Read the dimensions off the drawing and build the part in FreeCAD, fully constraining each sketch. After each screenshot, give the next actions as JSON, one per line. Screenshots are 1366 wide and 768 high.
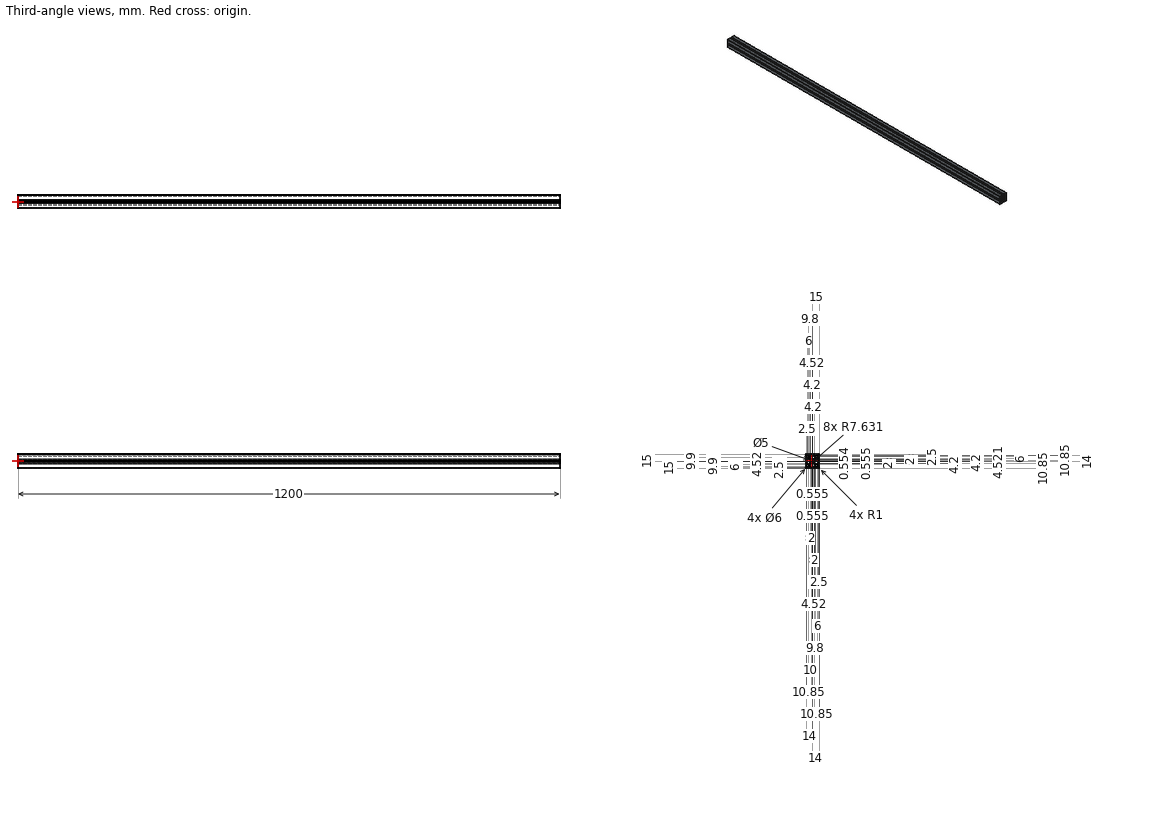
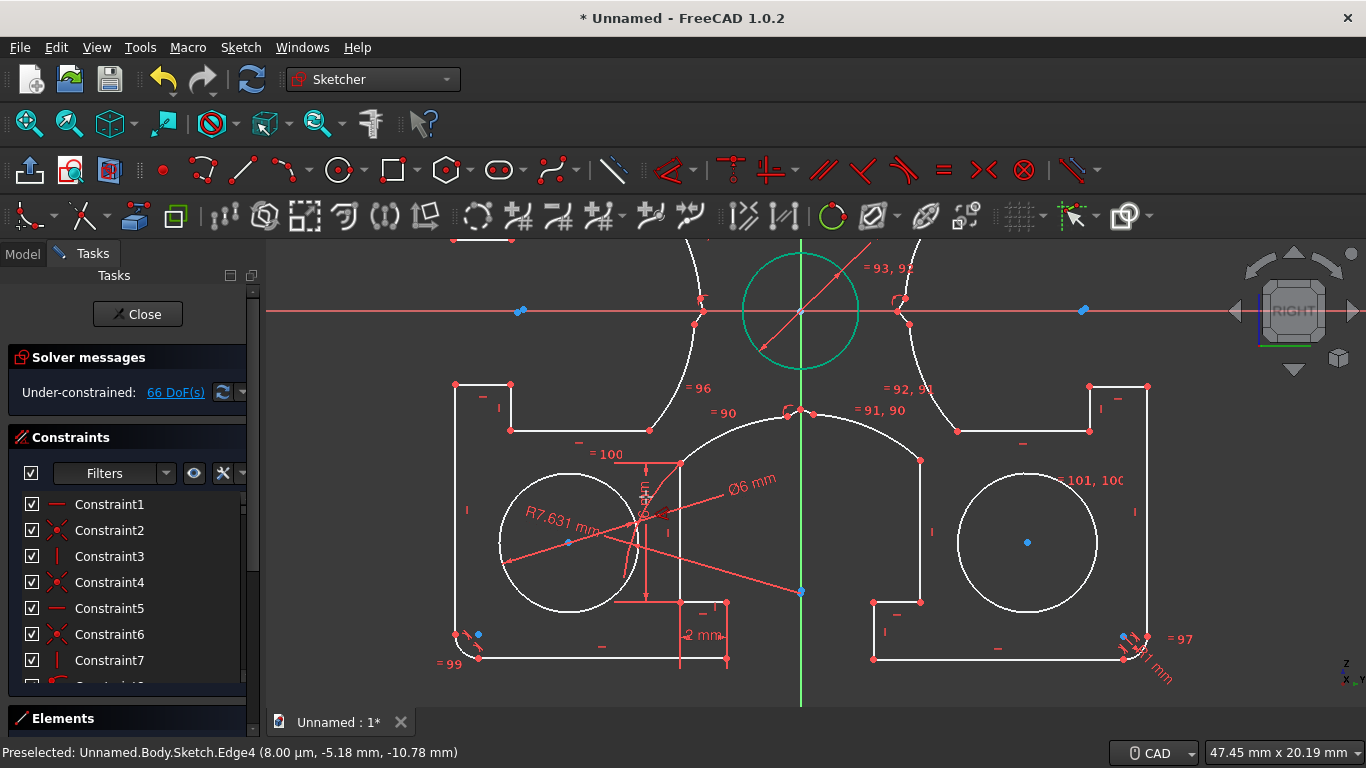
{"action": "left_click", "coordinate": [920, 503]}
{"action": "left_click", "coordinate": [954, 499]}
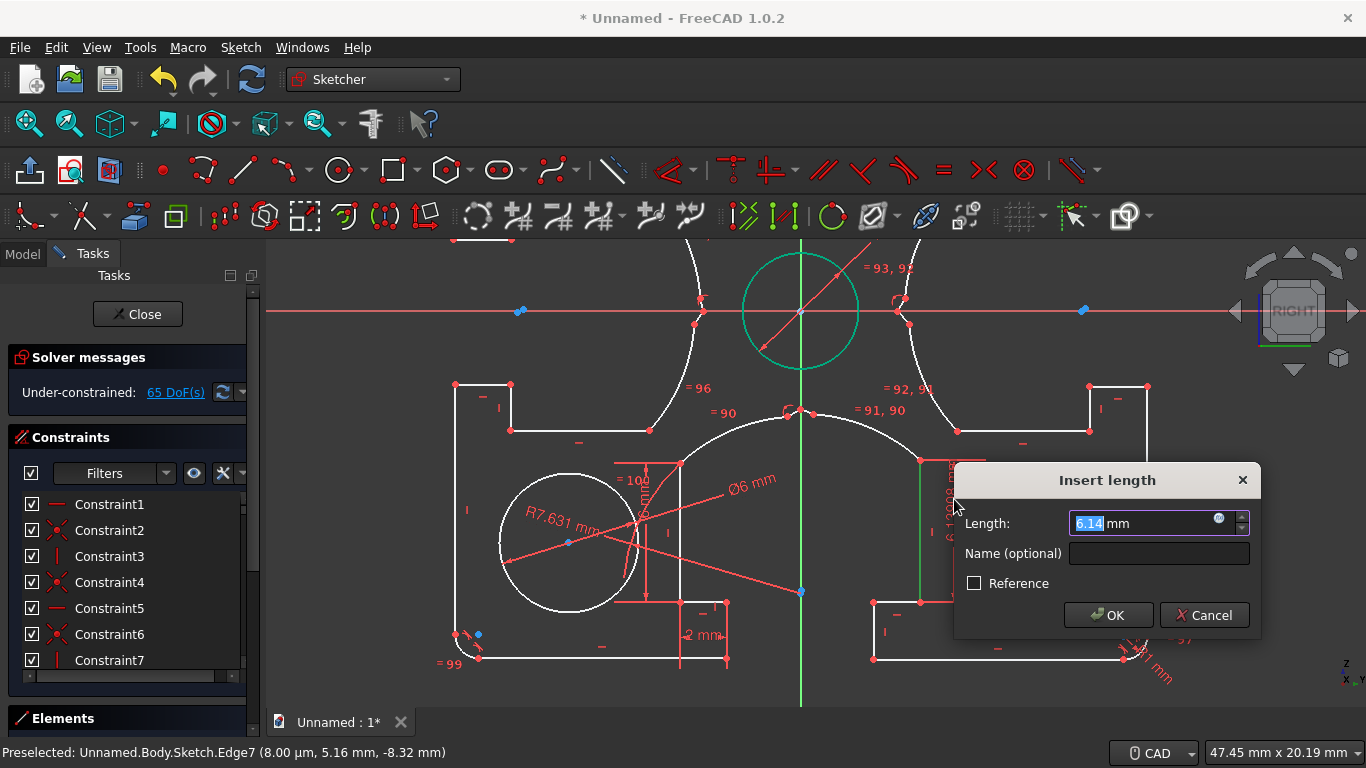
{"action": "type", "text": "6"}
{"action": "key", "text": "Return"}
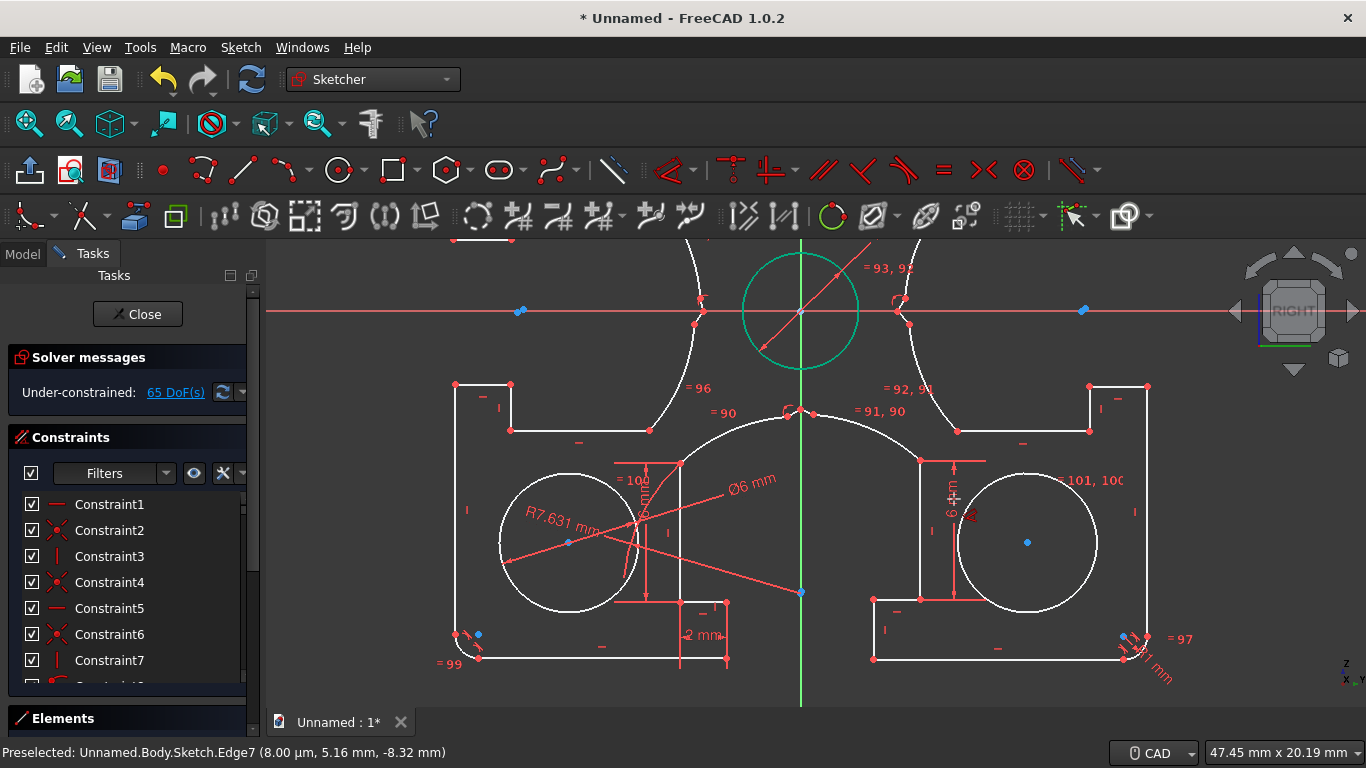
{"action": "left_click", "coordinate": [906, 600]}
{"action": "left_click", "coordinate": [897, 634]}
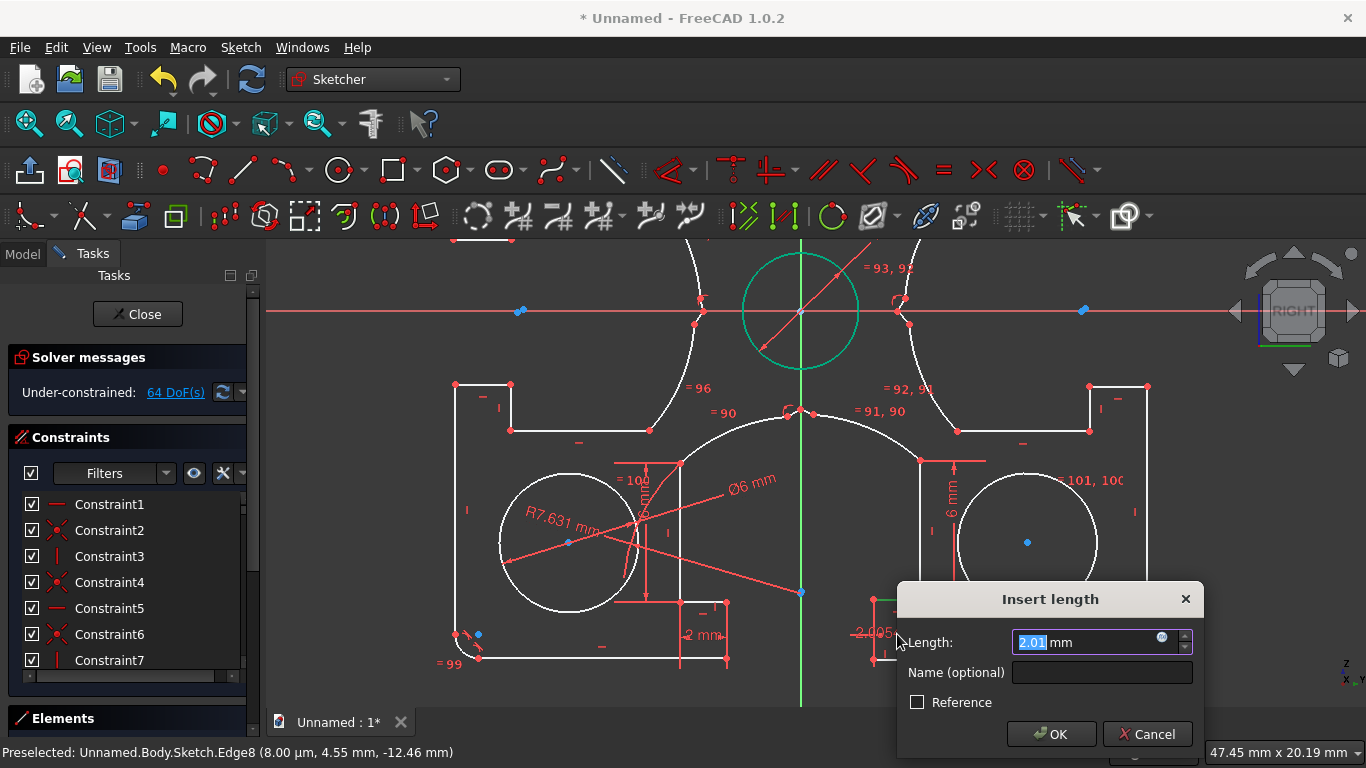
{"action": "type", "text": "2"}
{"action": "key", "text": "Return"}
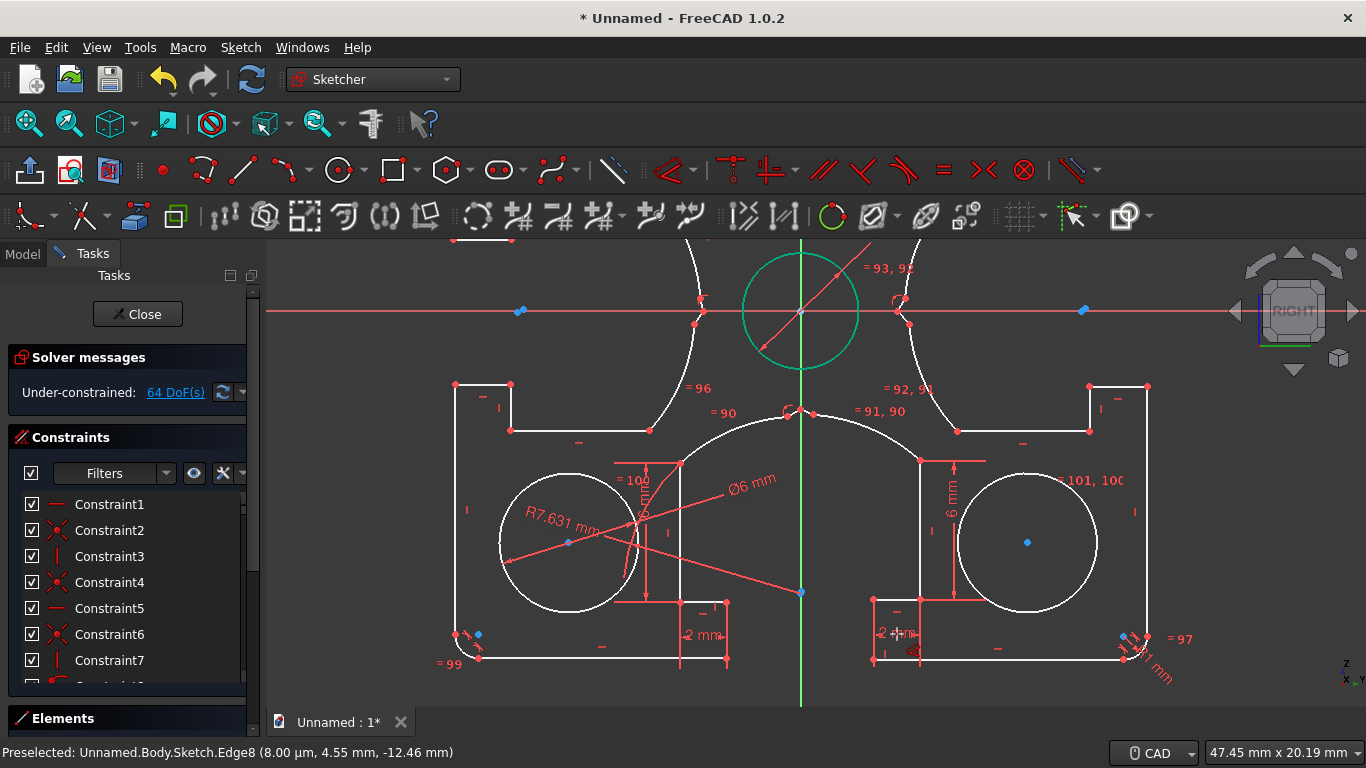
{"action": "left_click", "coordinate": [1090, 400]}
{"action": "left_click", "coordinate": [1124, 409]}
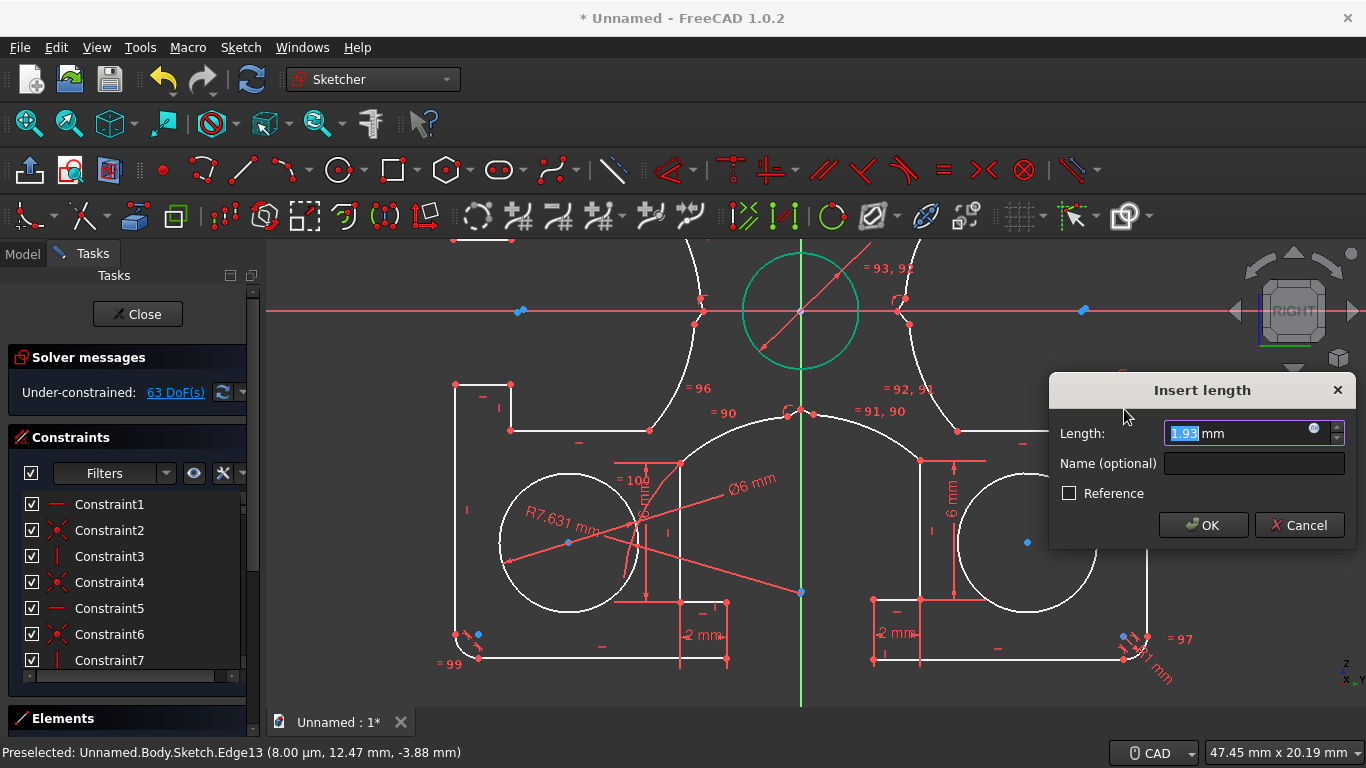
{"action": "type", "text": "2"}
{"action": "key", "text": "Return"}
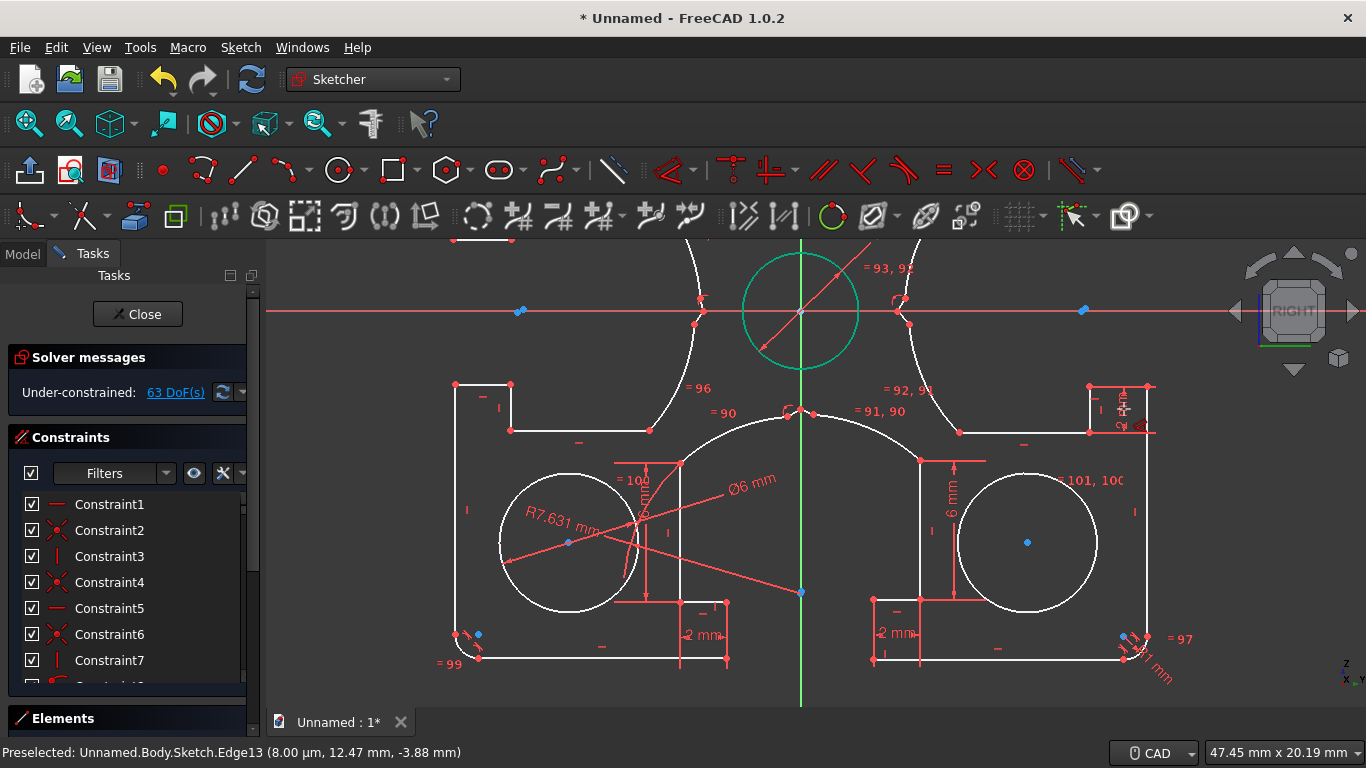
{"action": "left_click", "coordinate": [1051, 433]}
{"action": "left_click", "coordinate": [994, 467]}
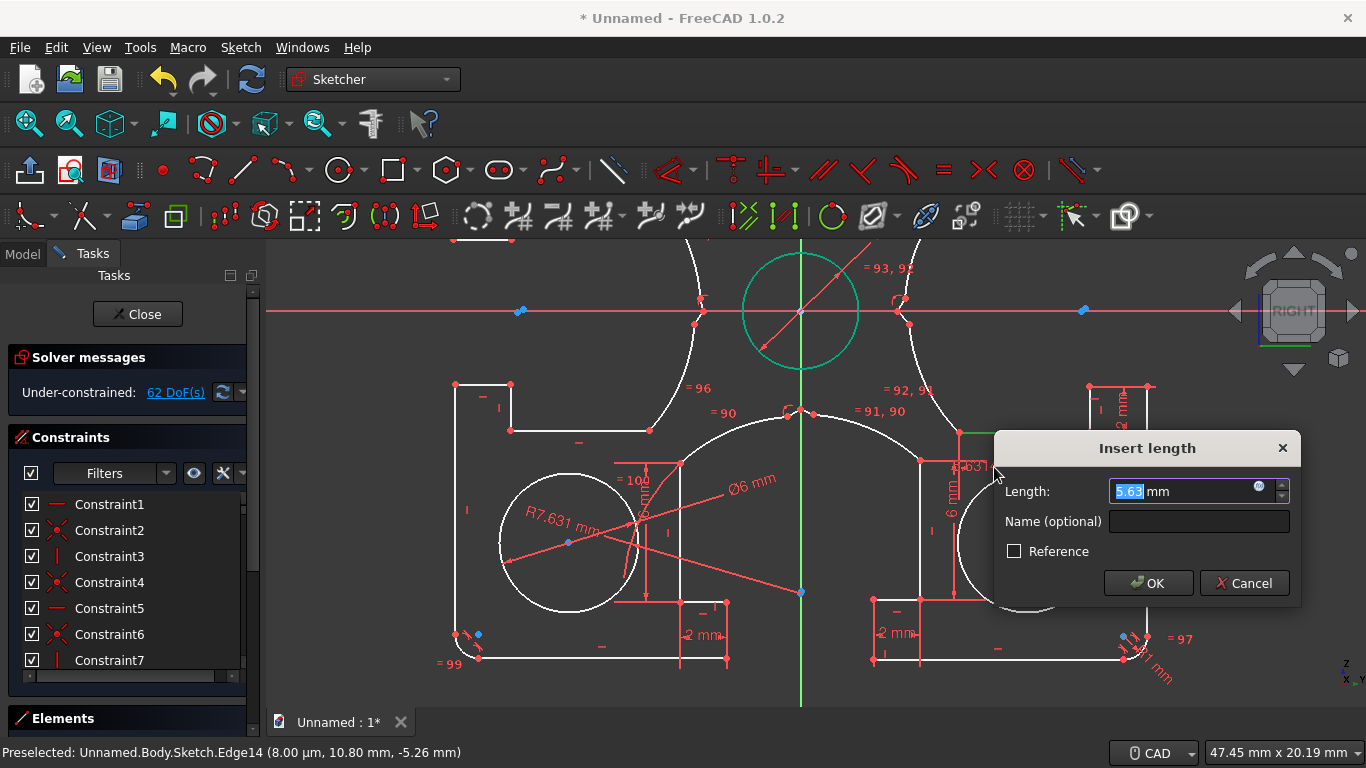
{"action": "type", "text": "6"}
{"action": "key", "text": "Return"}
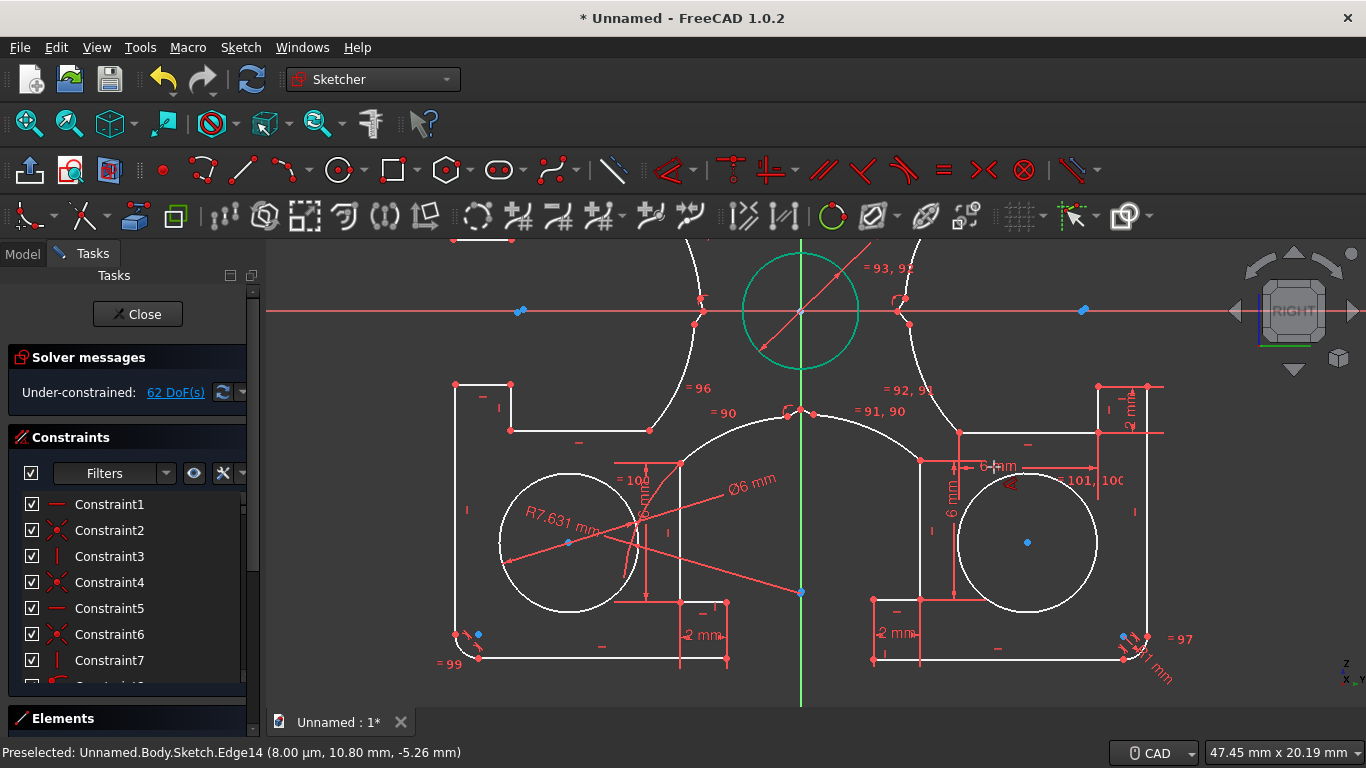
{"action": "scroll", "coordinate": [704, 605], "scroll_direction": "down", "scroll_amount": 4}